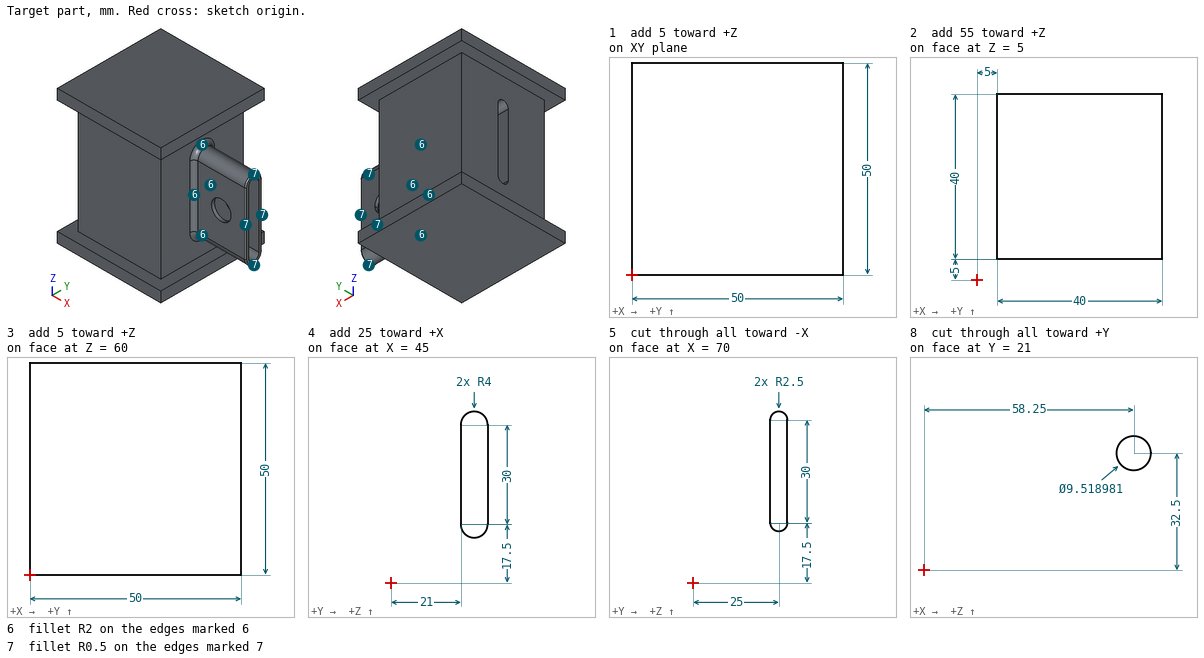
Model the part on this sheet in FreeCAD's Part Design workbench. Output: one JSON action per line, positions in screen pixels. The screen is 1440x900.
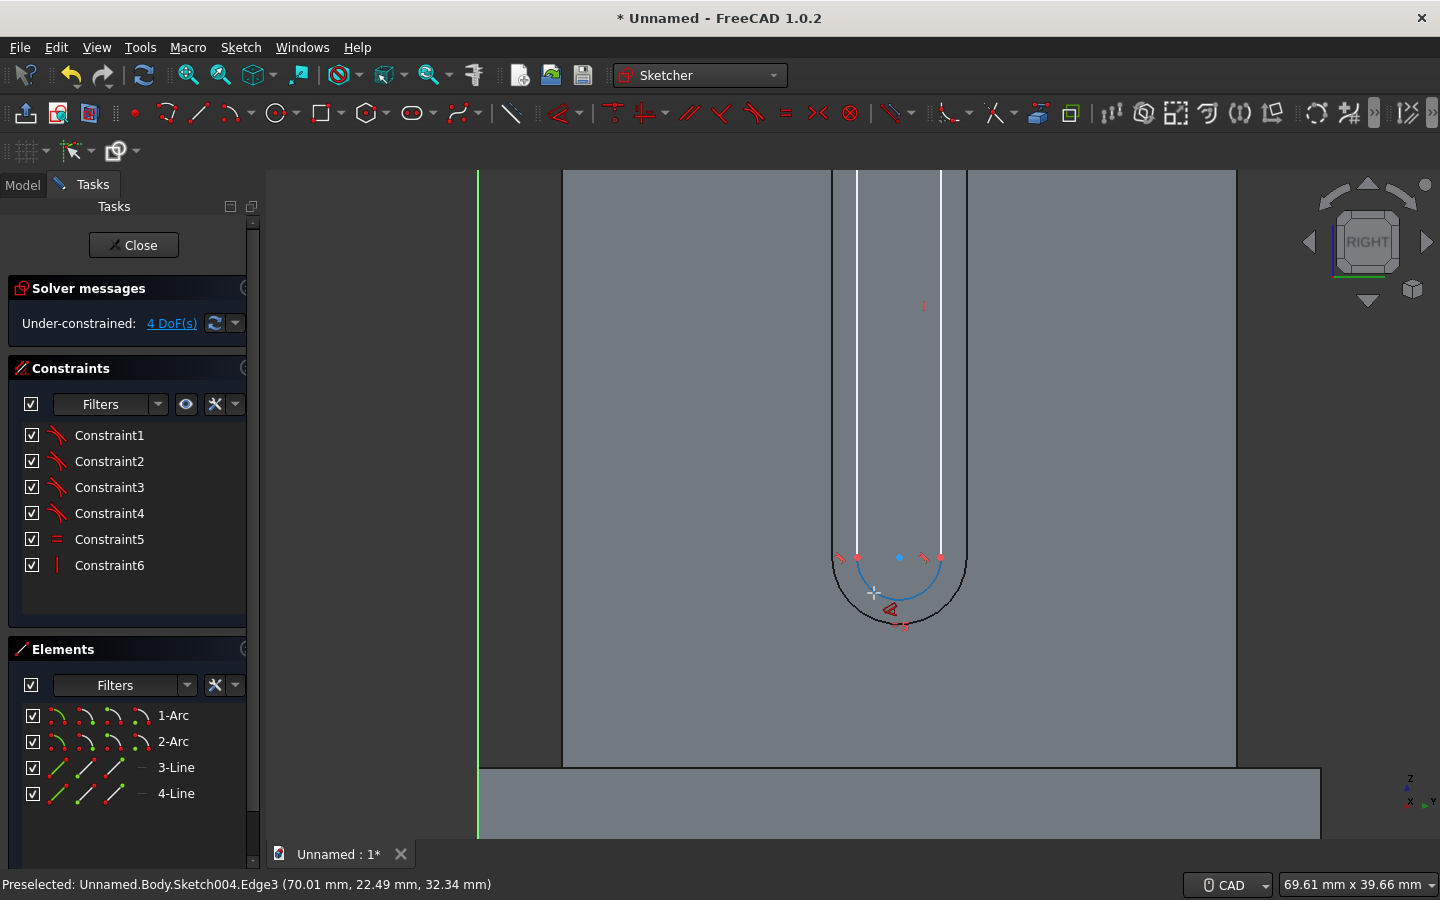
{"action": "left_click", "coordinate": [874, 592]}
{"action": "left_click", "coordinate": [855, 618]}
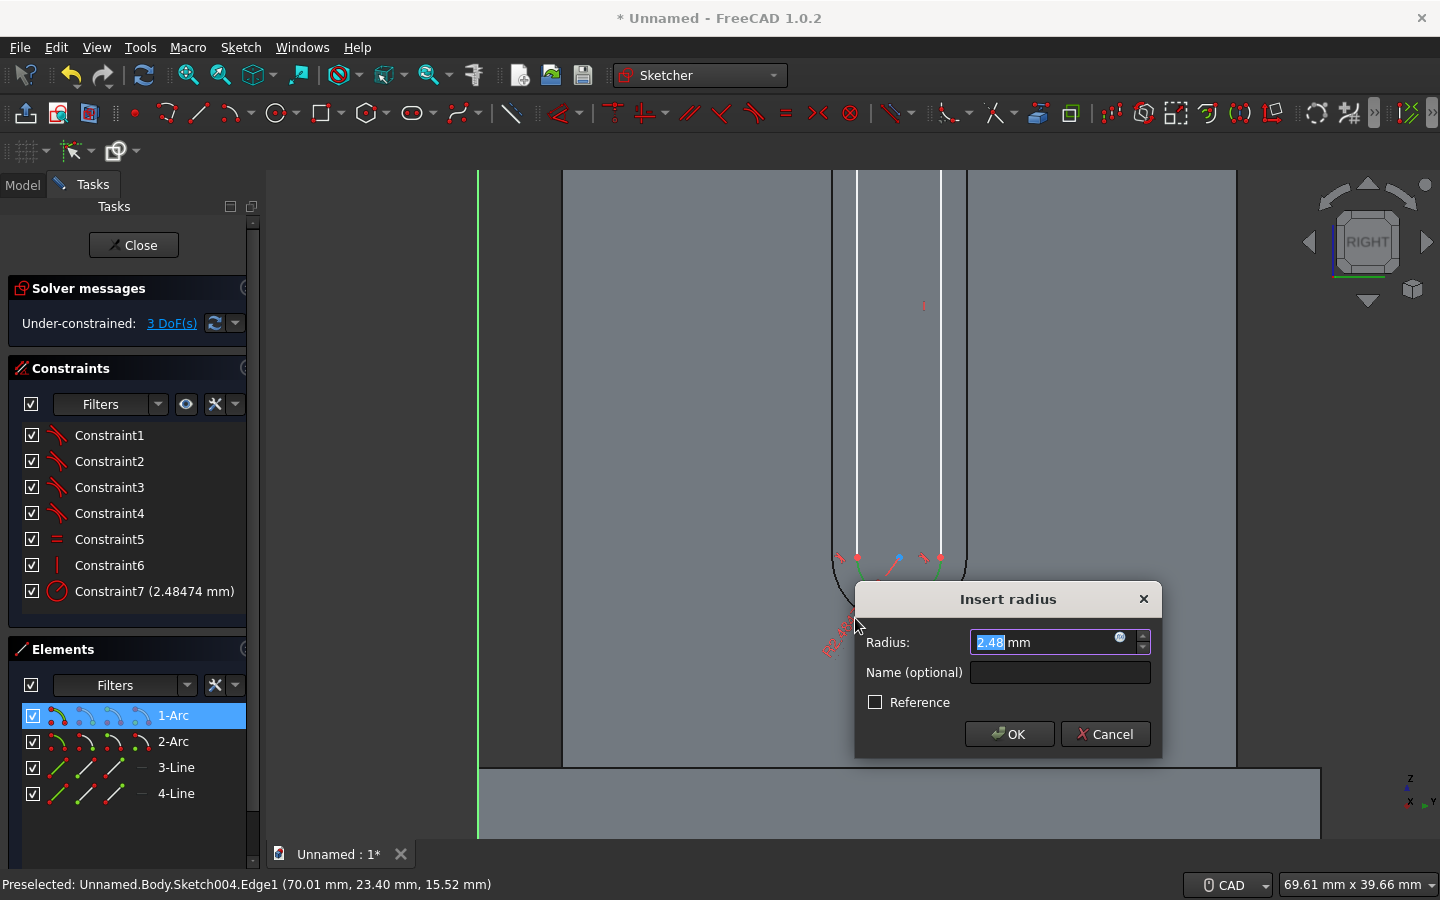
{"action": "type", "text": "2.5"}
{"action": "key", "text": "Return"}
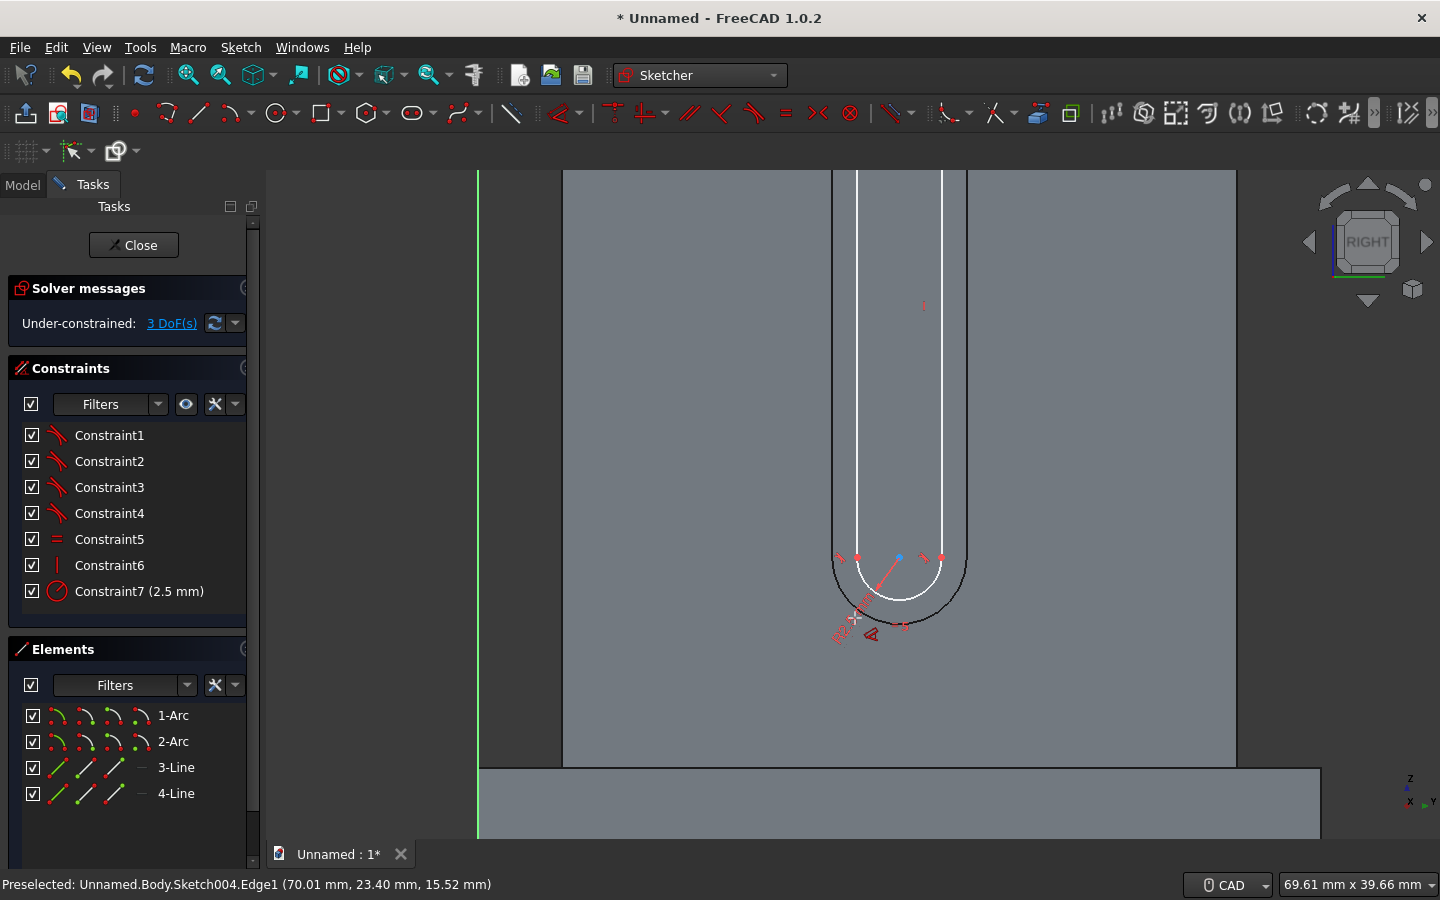
{"action": "left_click", "coordinate": [857, 406]}
{"action": "left_click", "coordinate": [891, 378]}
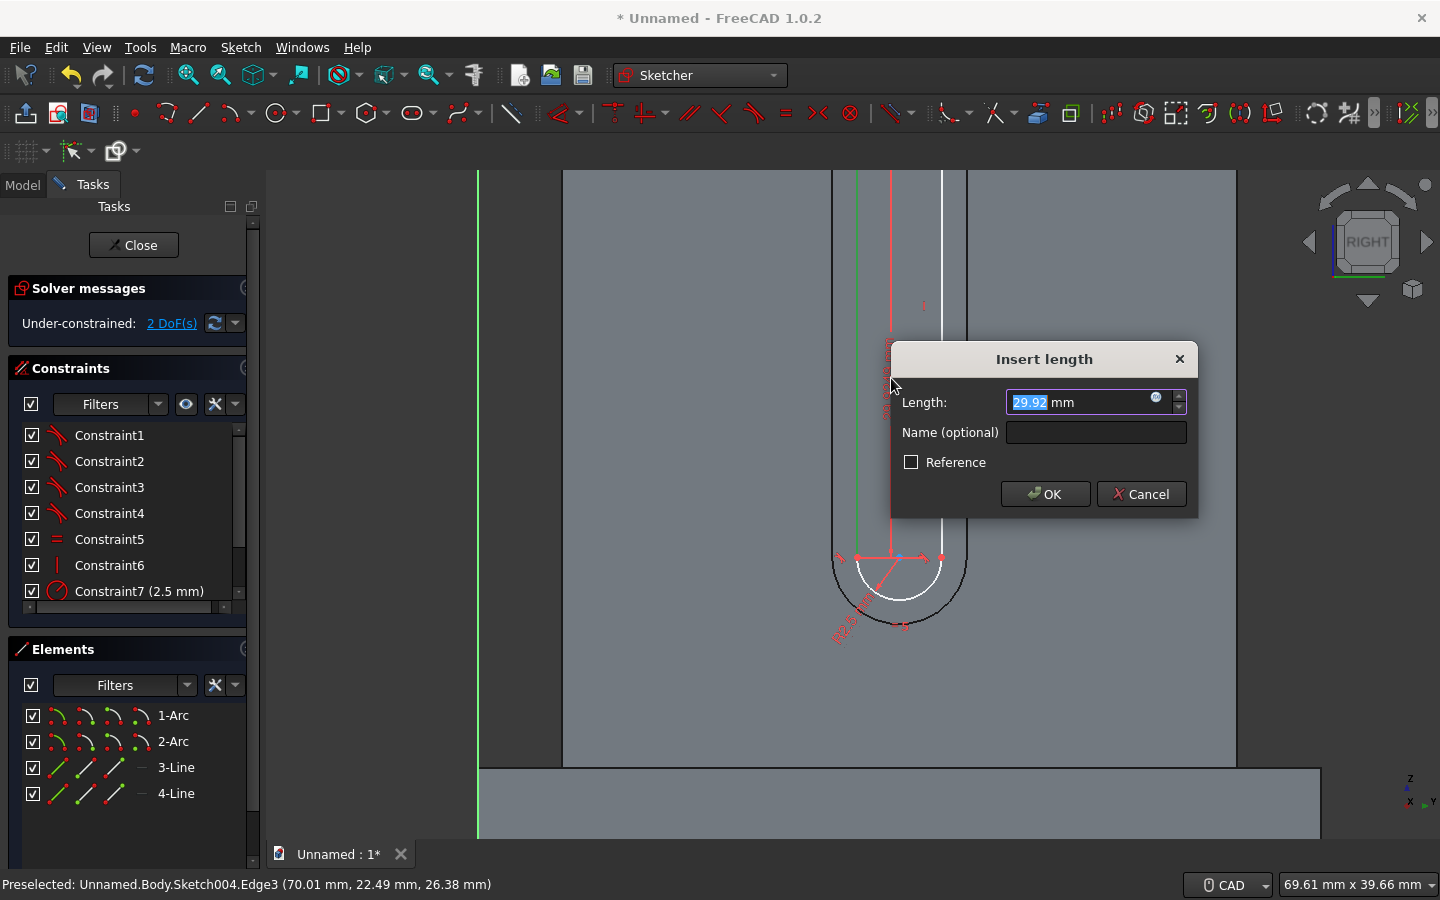
{"action": "type", "text": "30"}
{"action": "key", "text": "Return"}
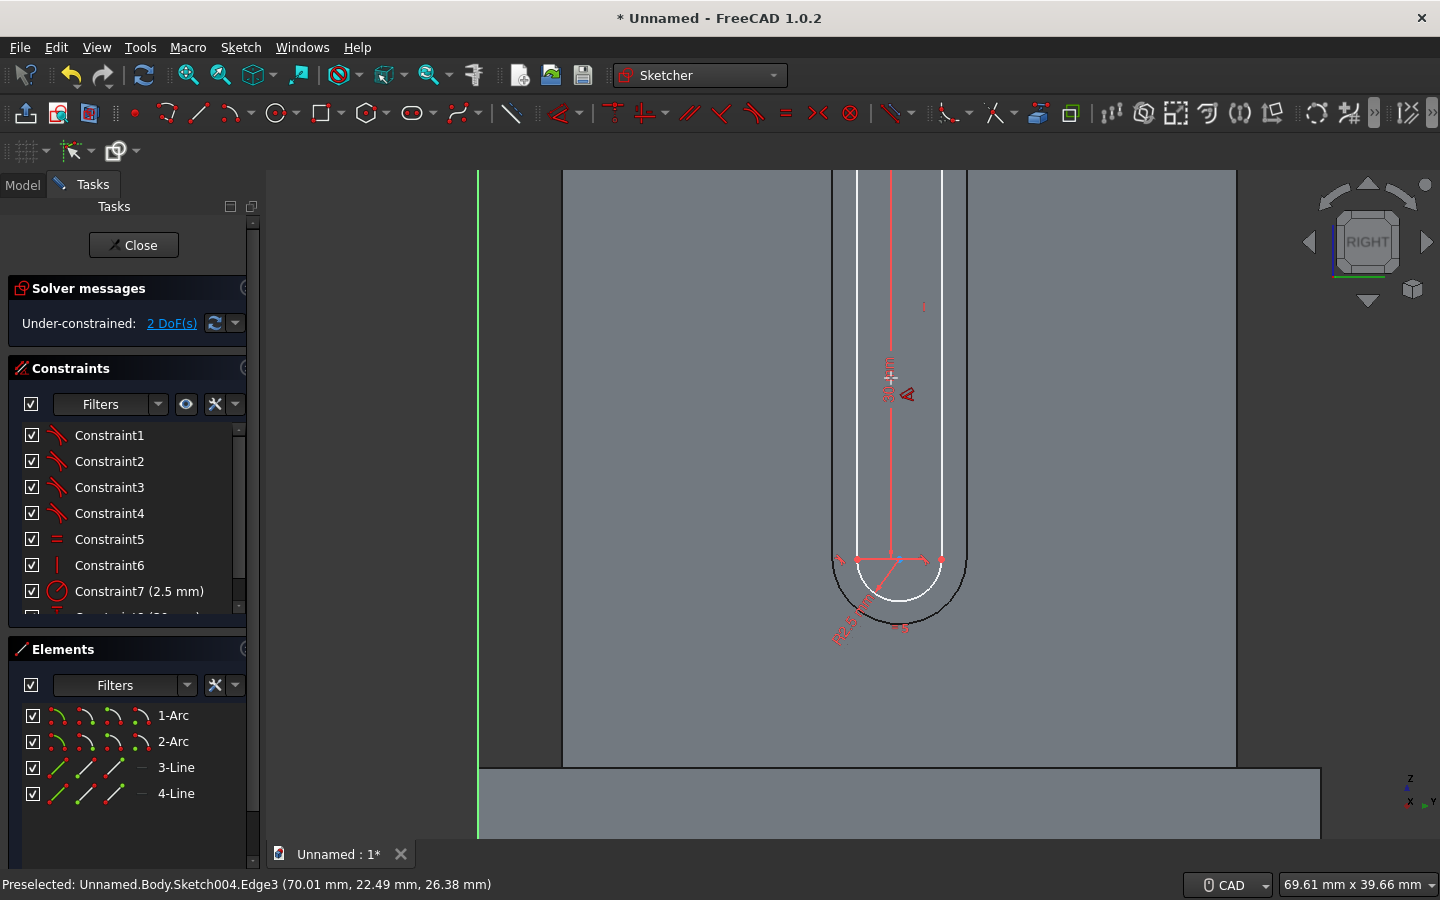
{"action": "left_click", "coordinate": [899, 559]}
{"action": "left_click", "coordinate": [689, 525]}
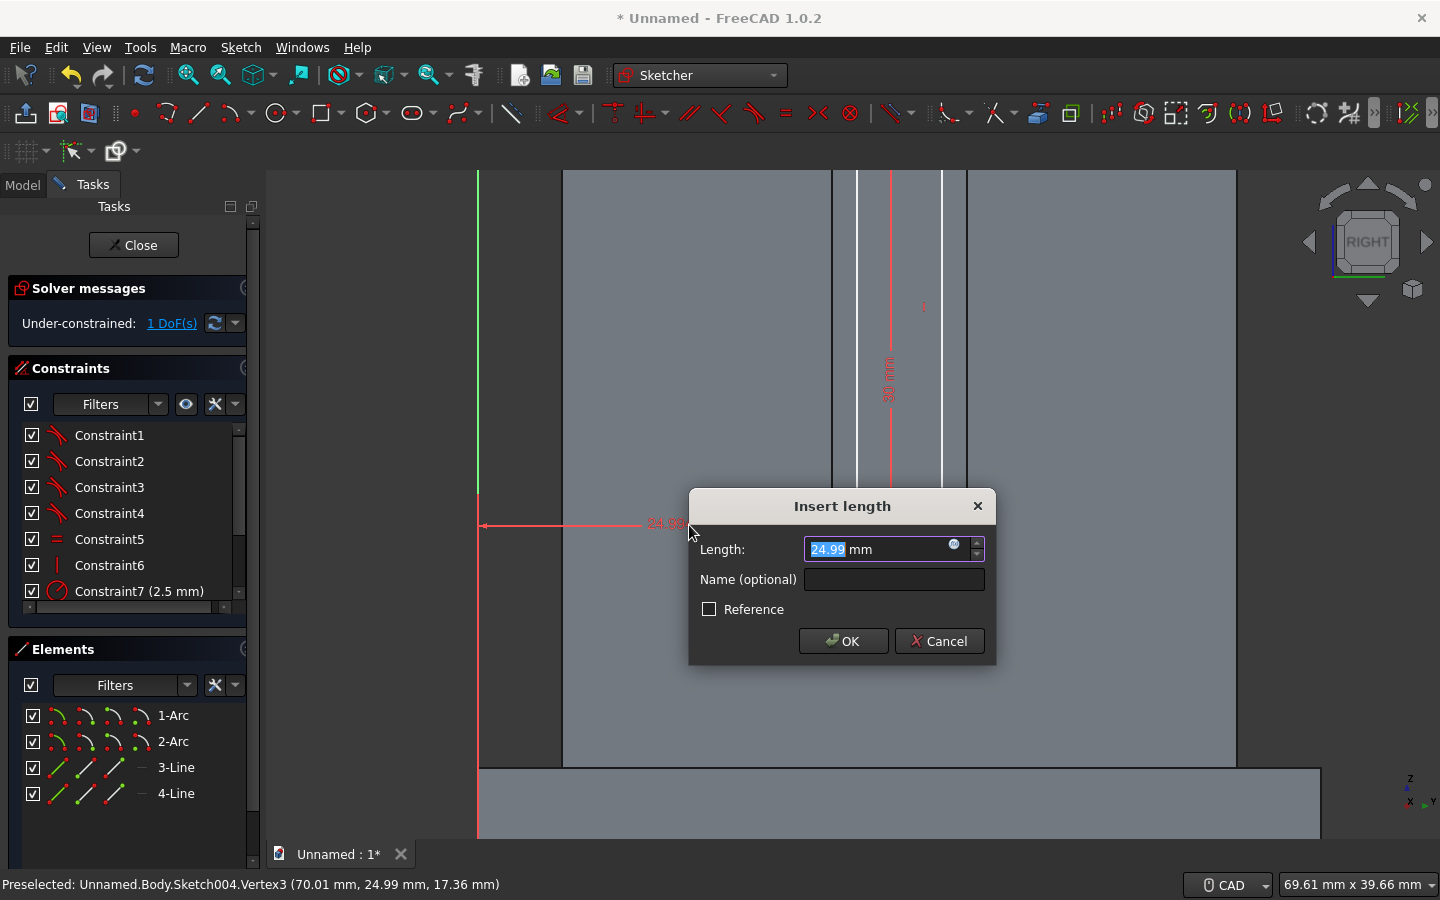
{"action": "type", "text": "25"}
{"action": "key", "text": "Return"}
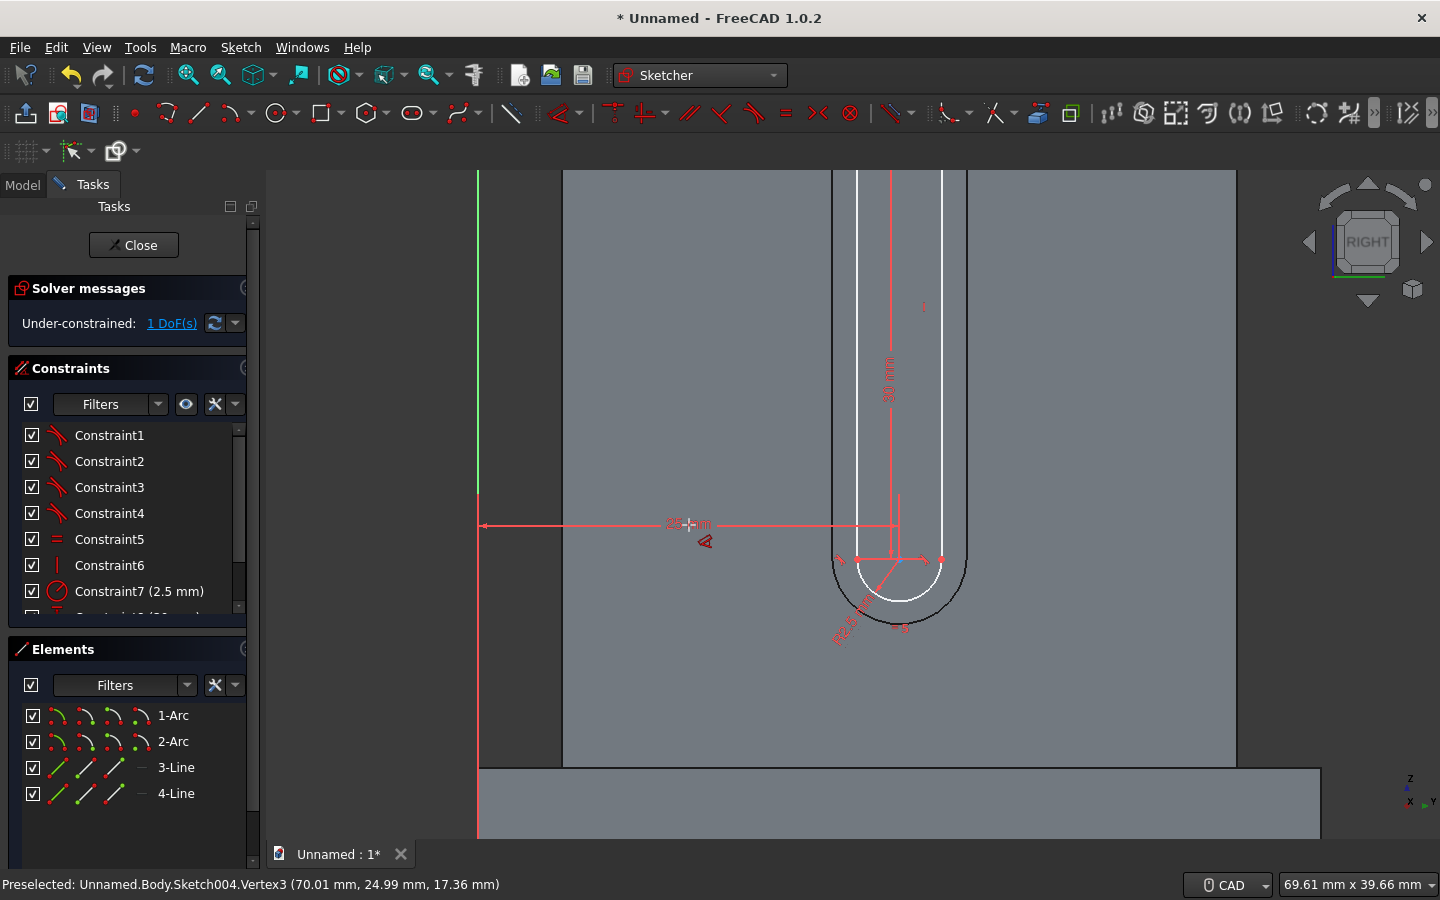
{"action": "left_click", "coordinate": [857, 559]}
{"action": "left_click", "coordinate": [444, 685]}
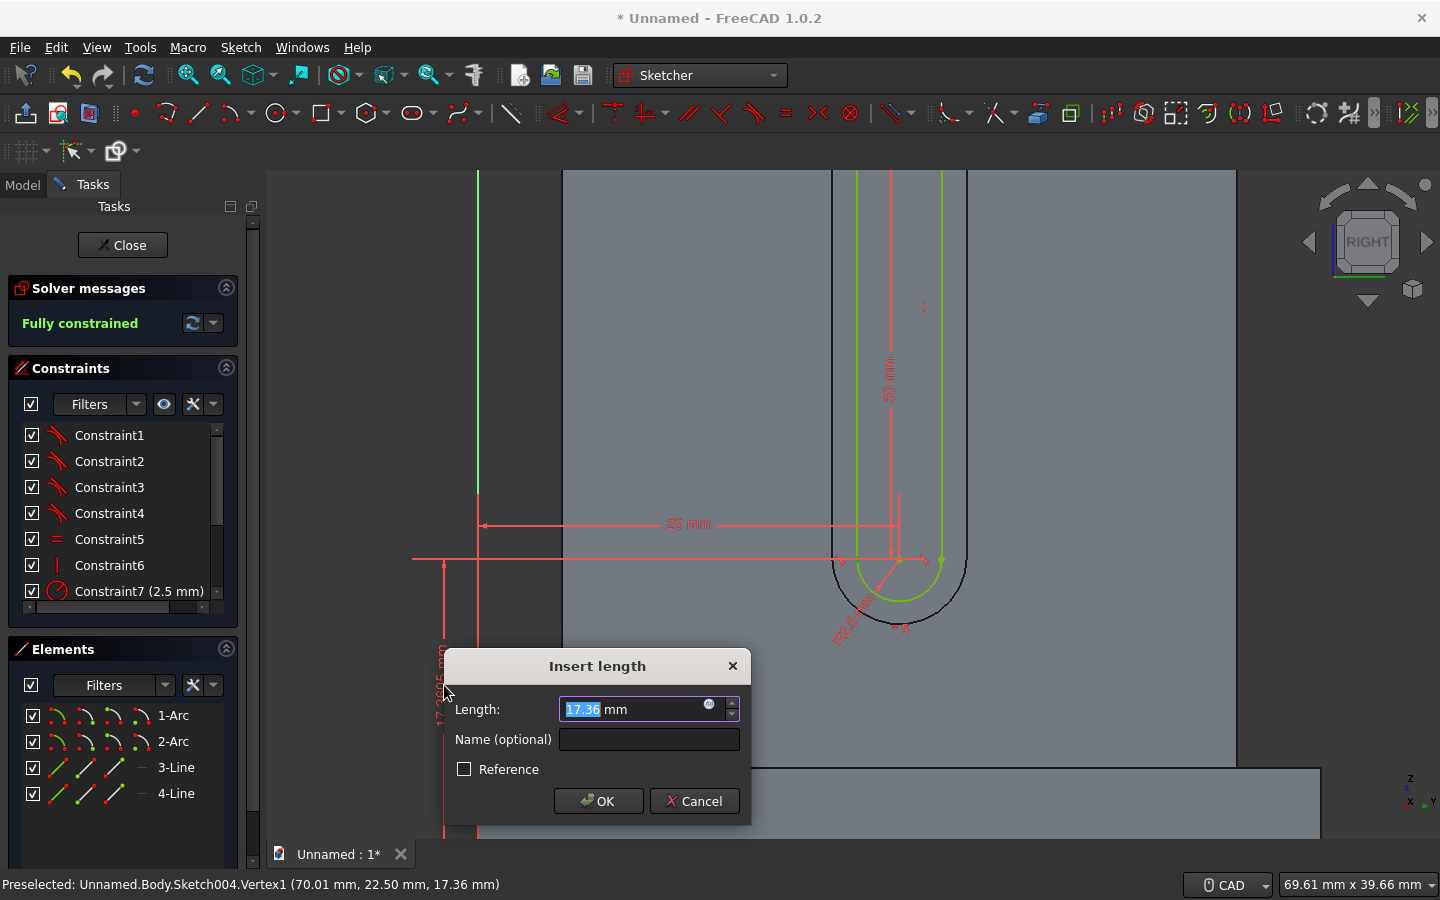
{"action": "type", "text": "17.5"}
{"action": "key", "text": "Return"}
{"action": "key", "text": "Escape"}